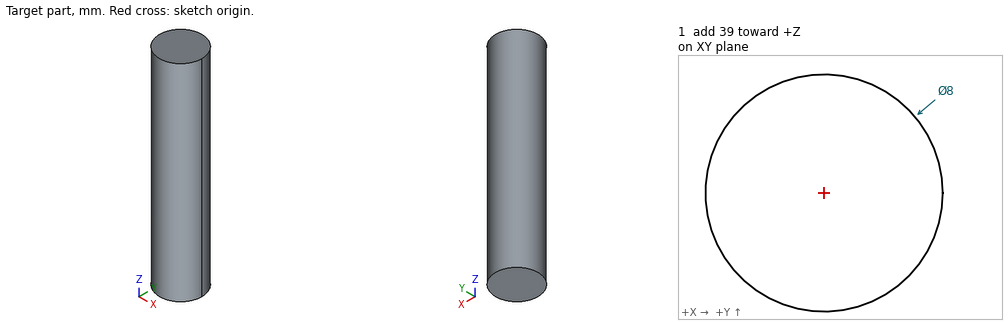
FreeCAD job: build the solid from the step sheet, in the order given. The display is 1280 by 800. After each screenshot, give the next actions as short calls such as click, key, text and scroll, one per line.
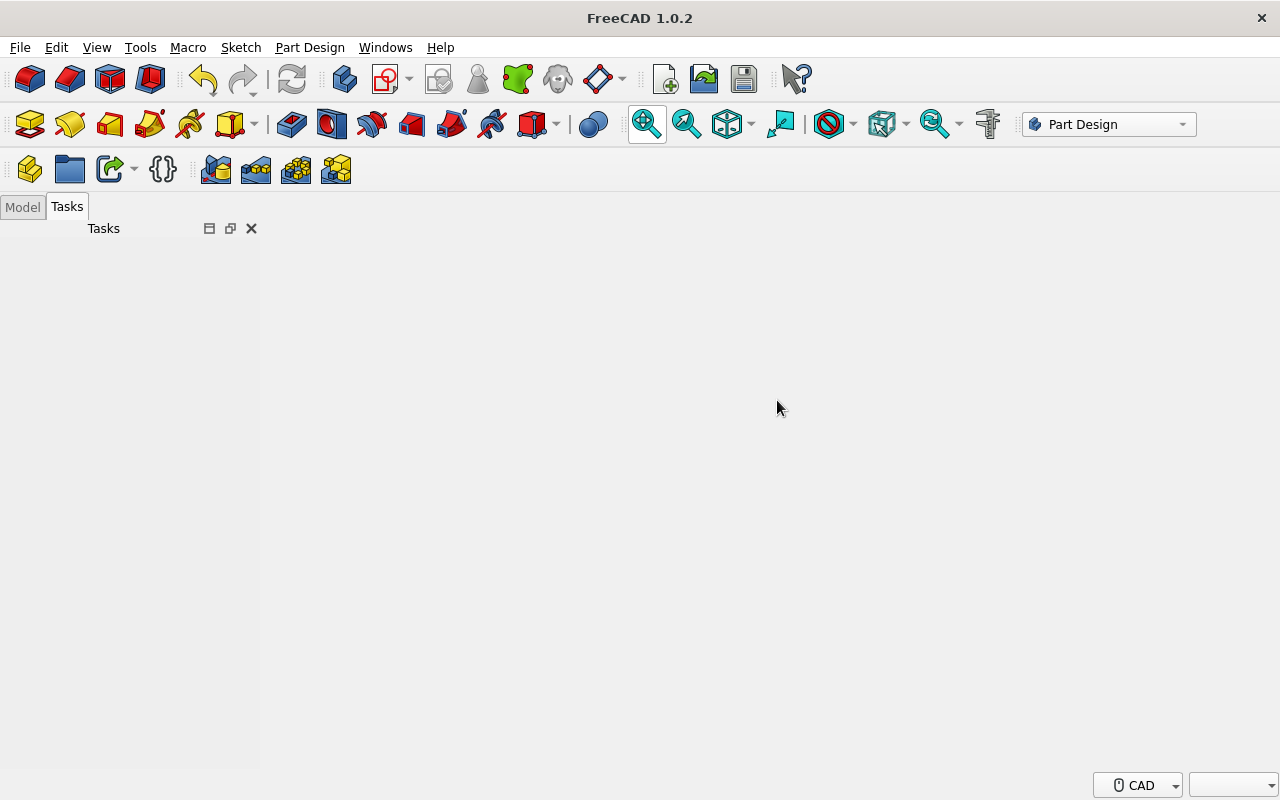
click(664, 80)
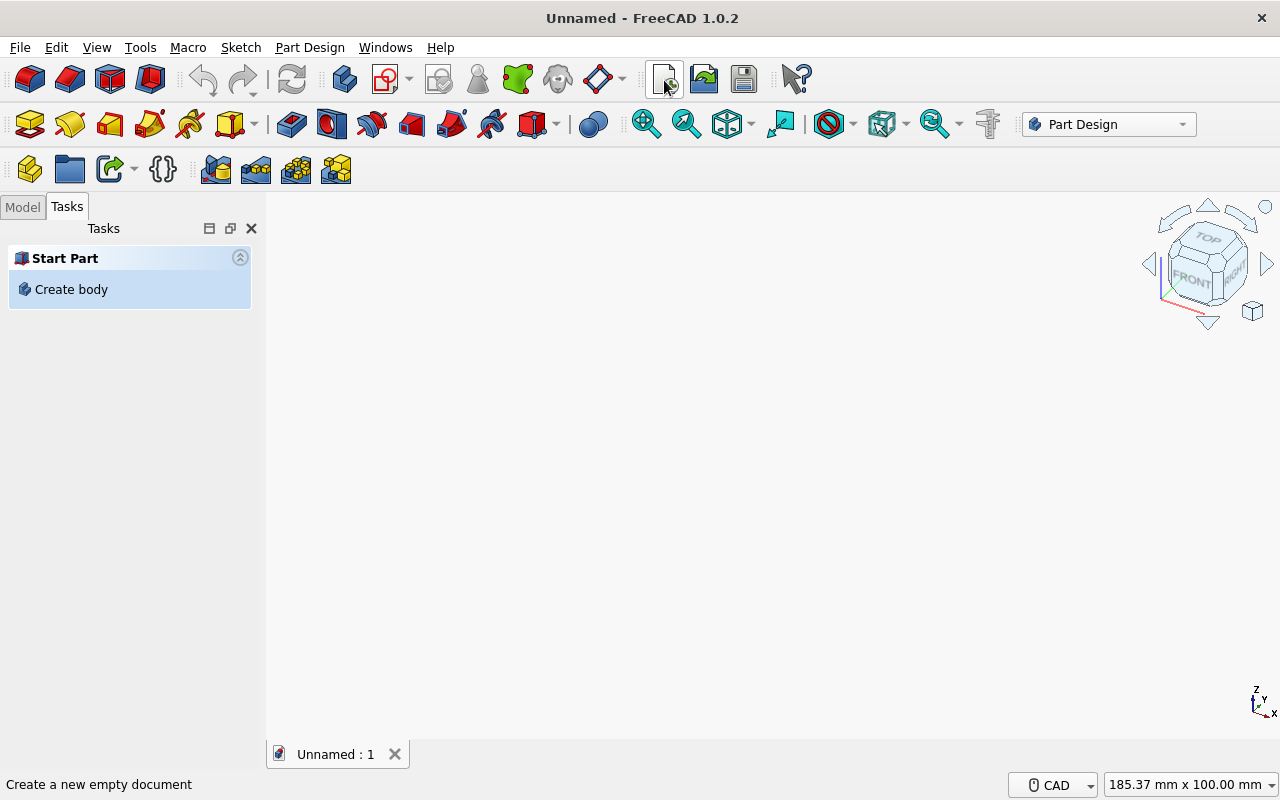
click(386, 80)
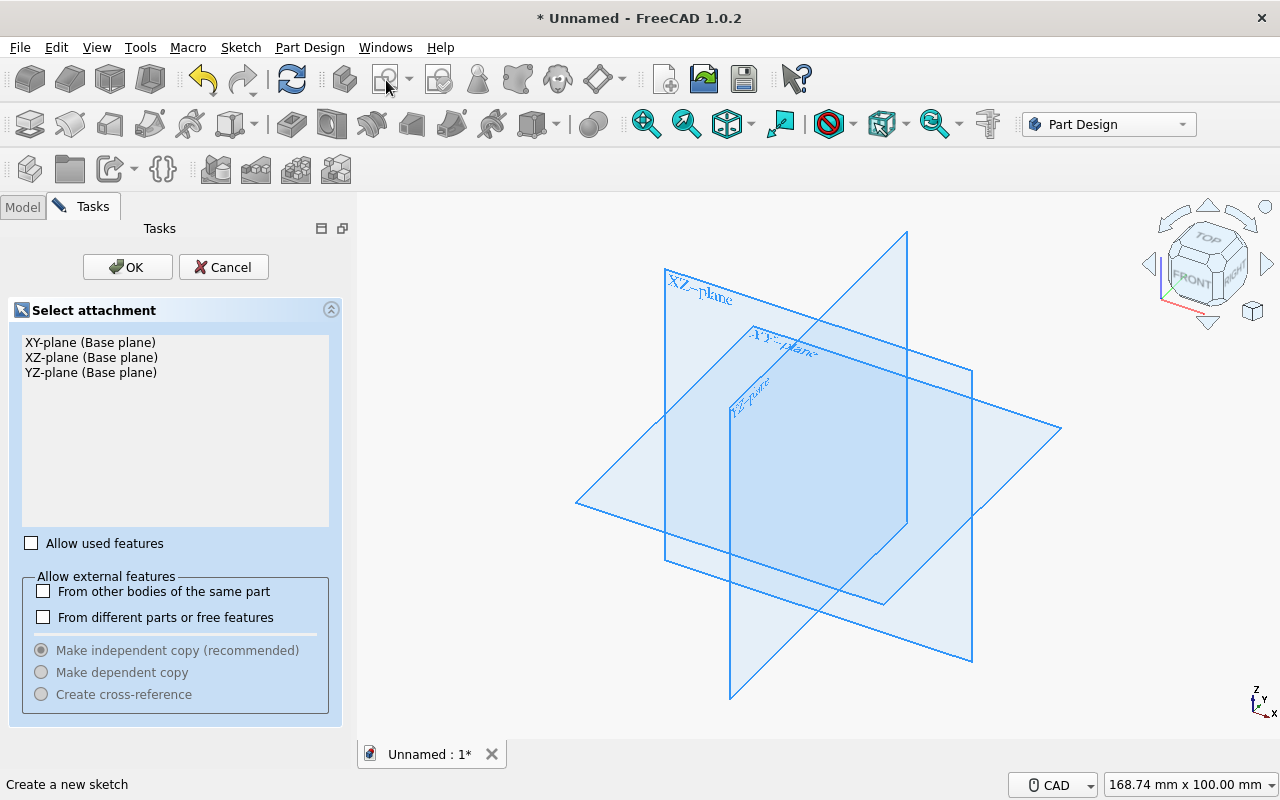
click(82, 342)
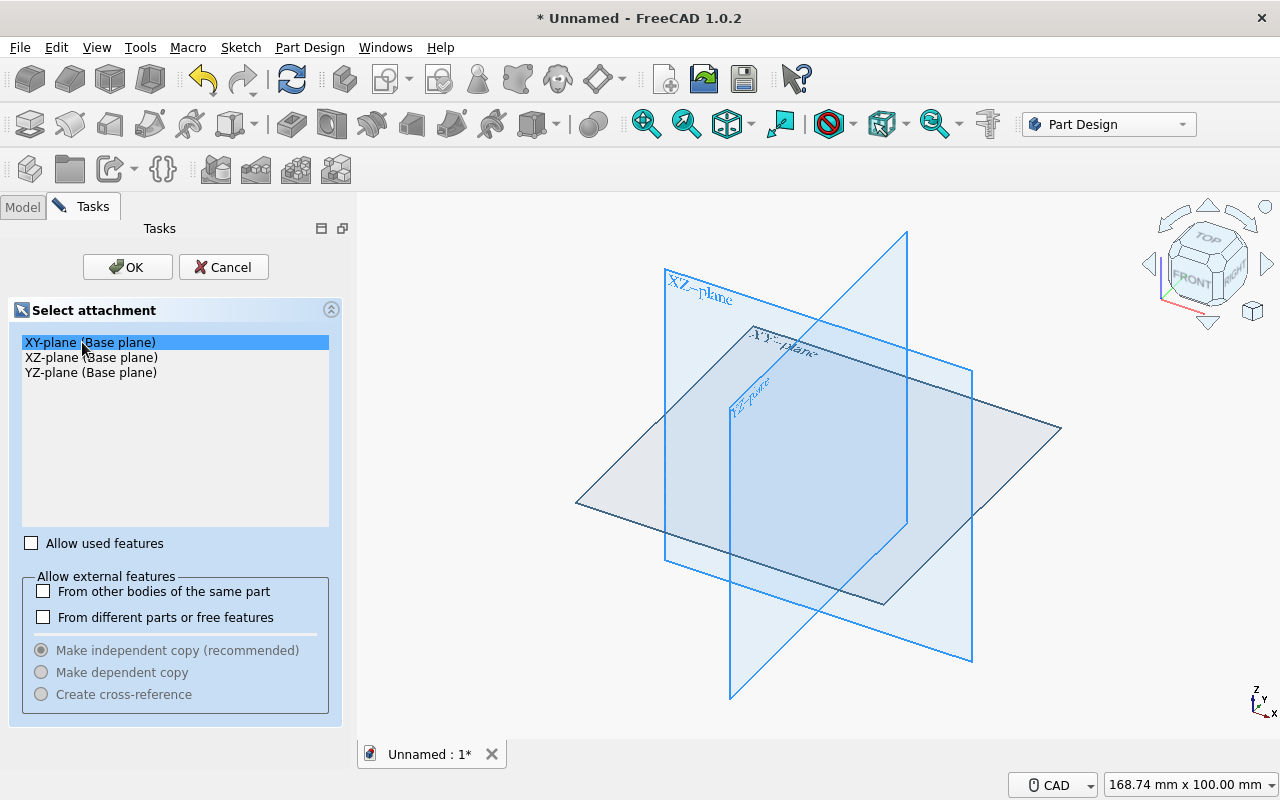
click(128, 267)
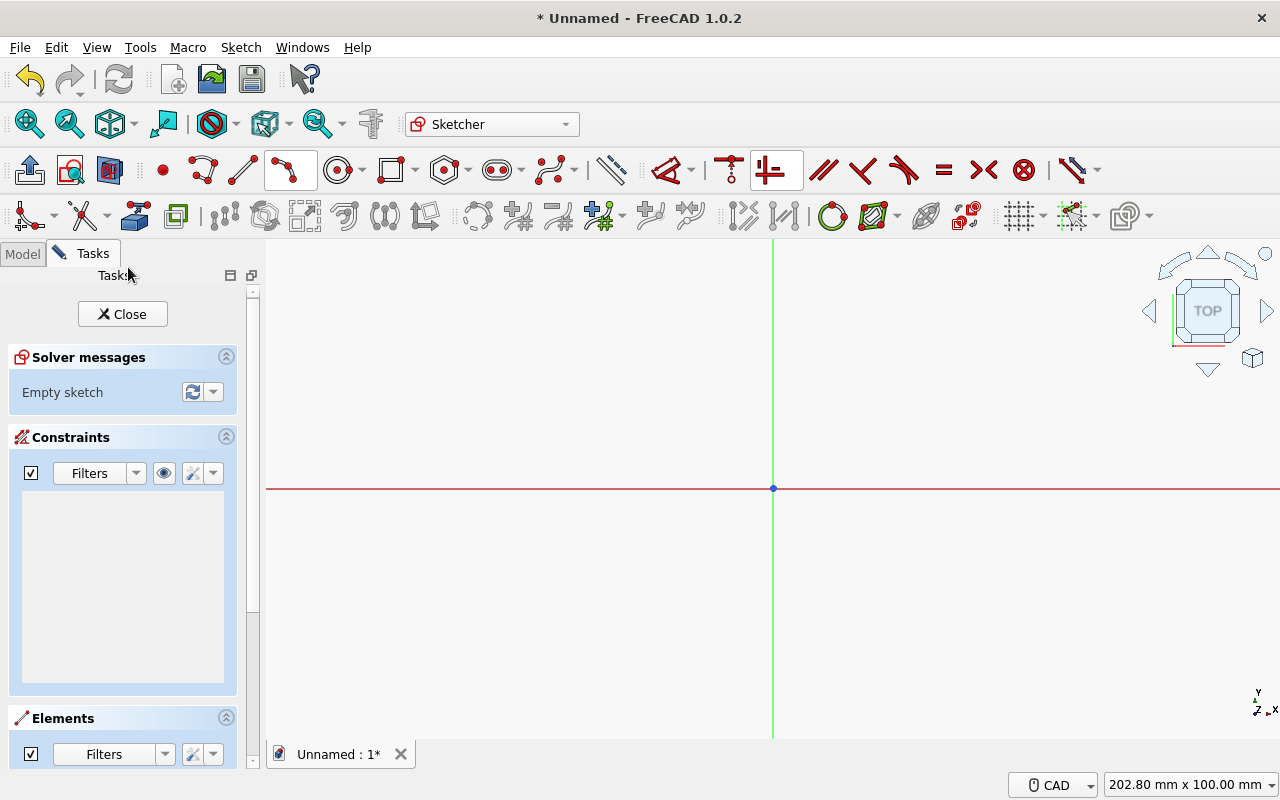
scroll(784, 489, up, 10)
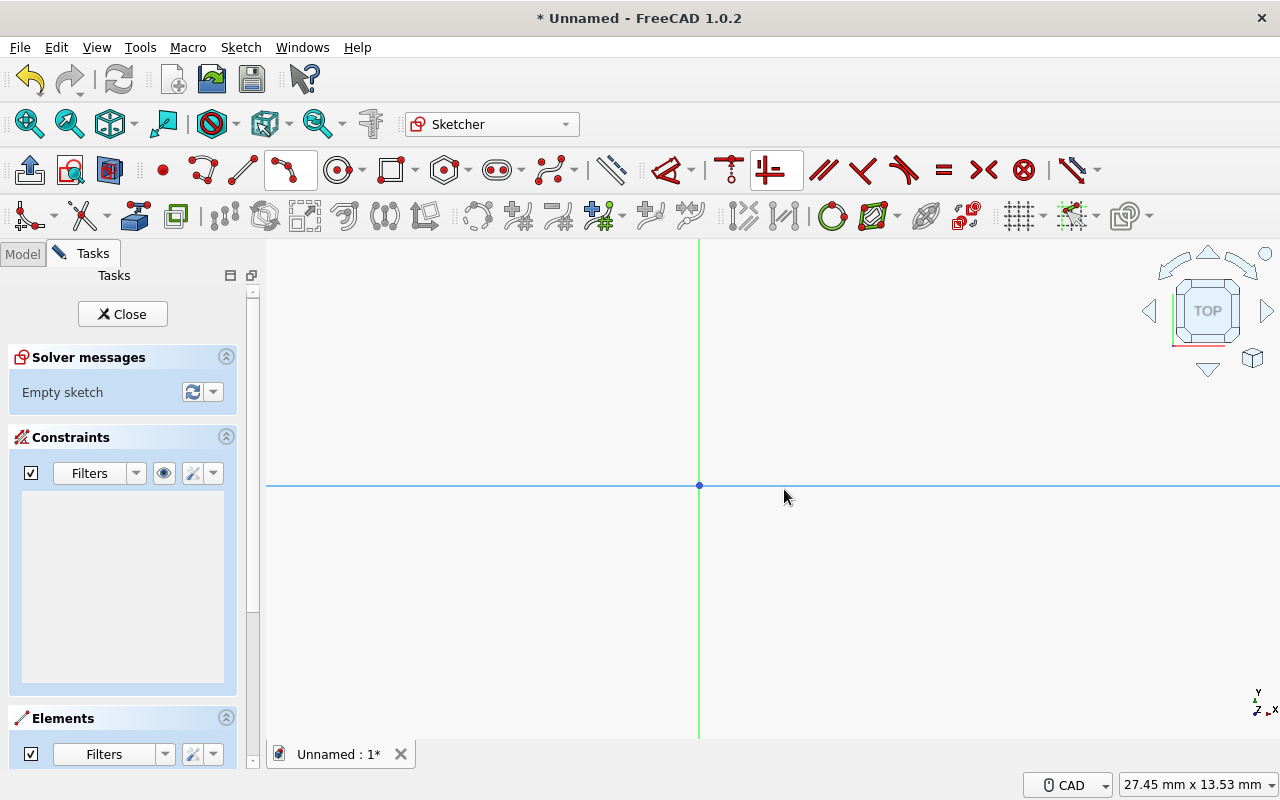
click(338, 170)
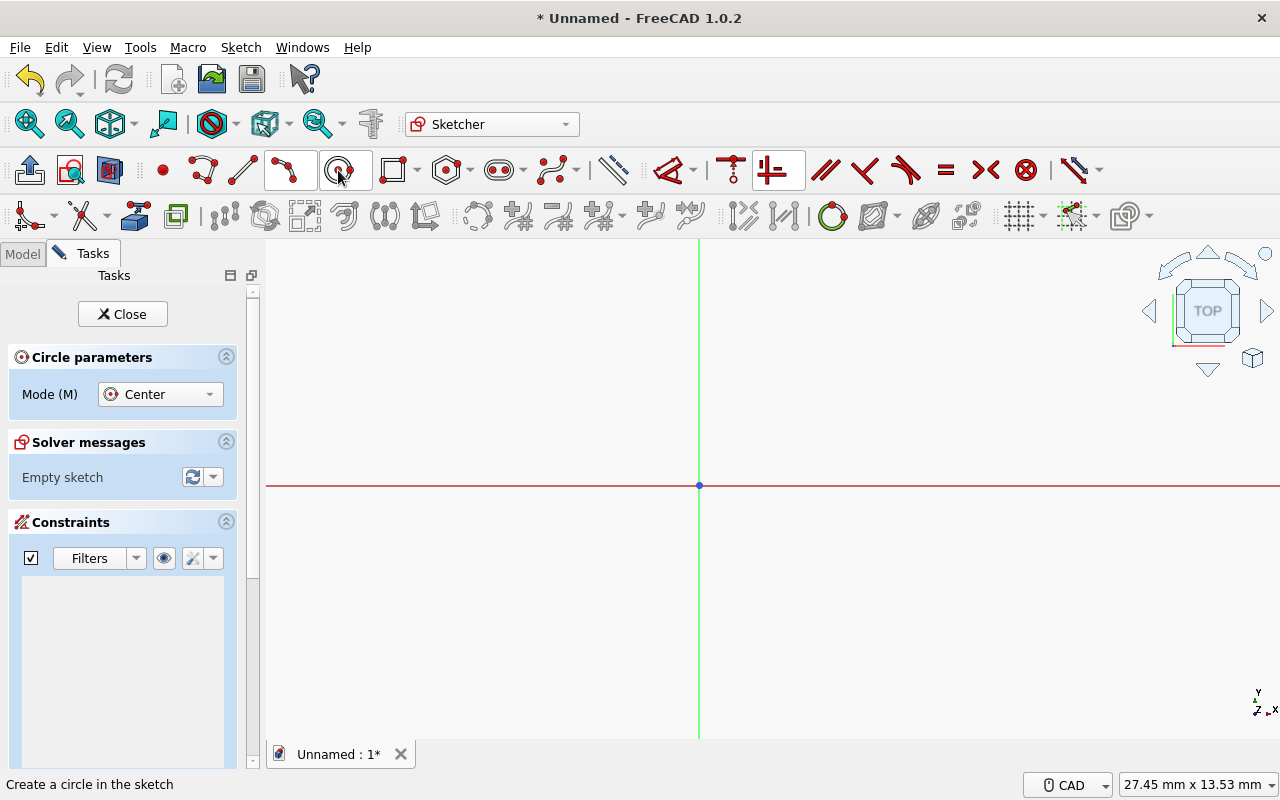
click(699, 486)
move(804, 381)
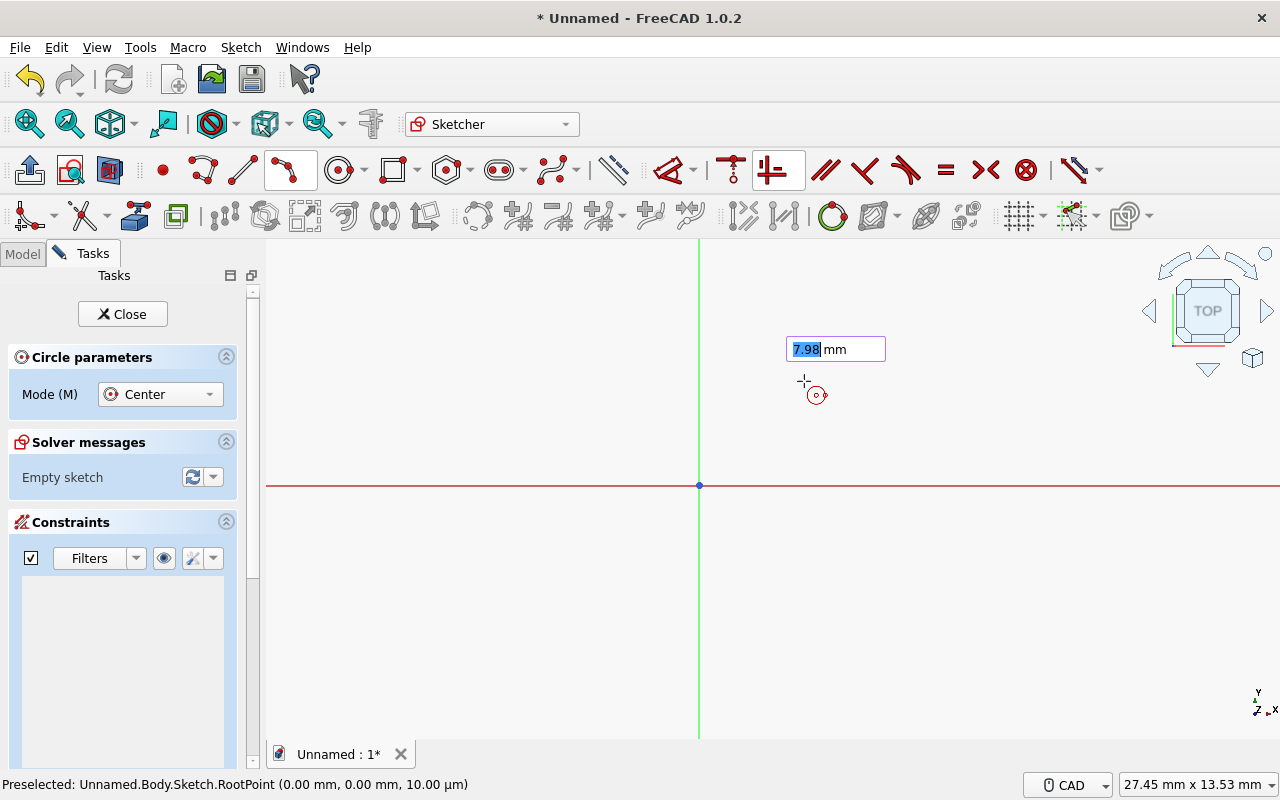
text(8)
key(Return)
key(Escape)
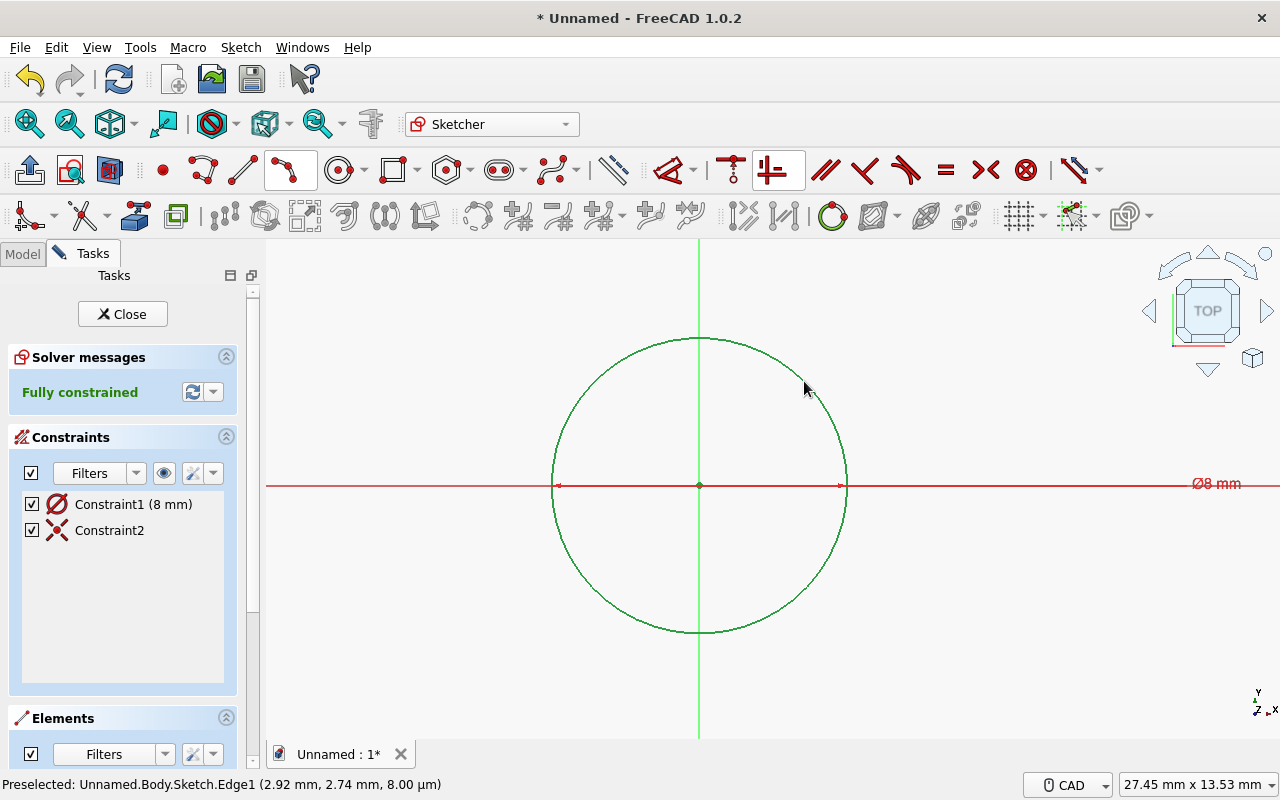
click(123, 314)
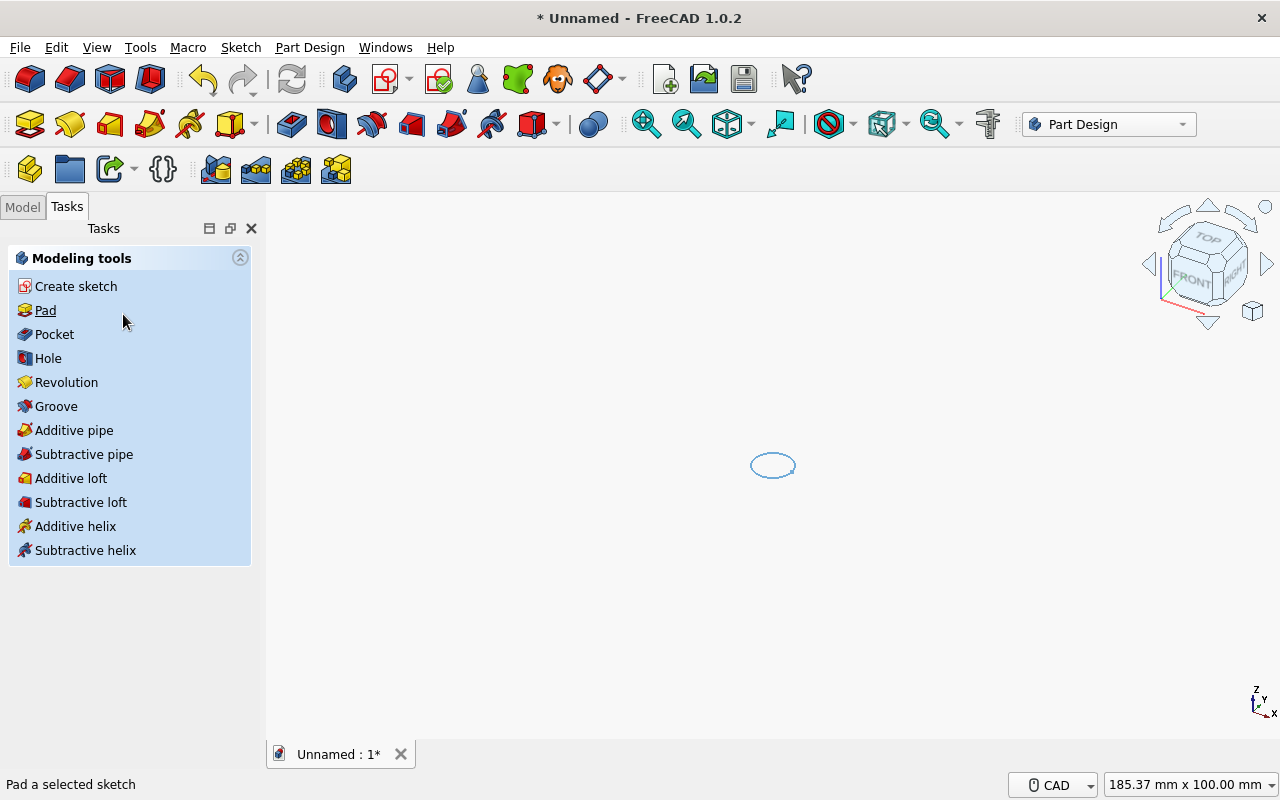
click(30, 124)